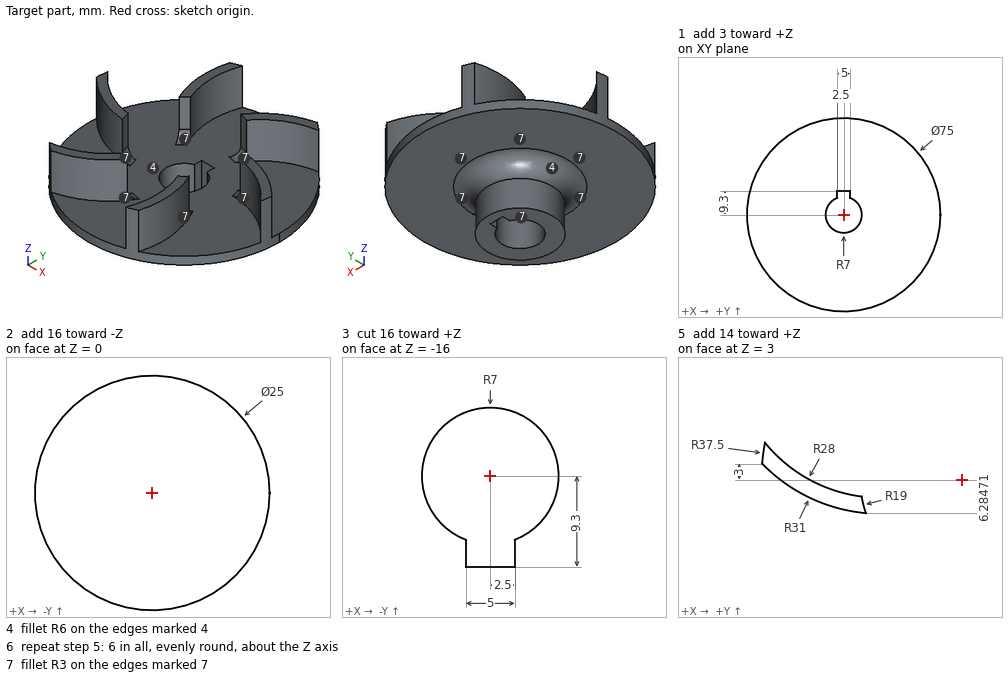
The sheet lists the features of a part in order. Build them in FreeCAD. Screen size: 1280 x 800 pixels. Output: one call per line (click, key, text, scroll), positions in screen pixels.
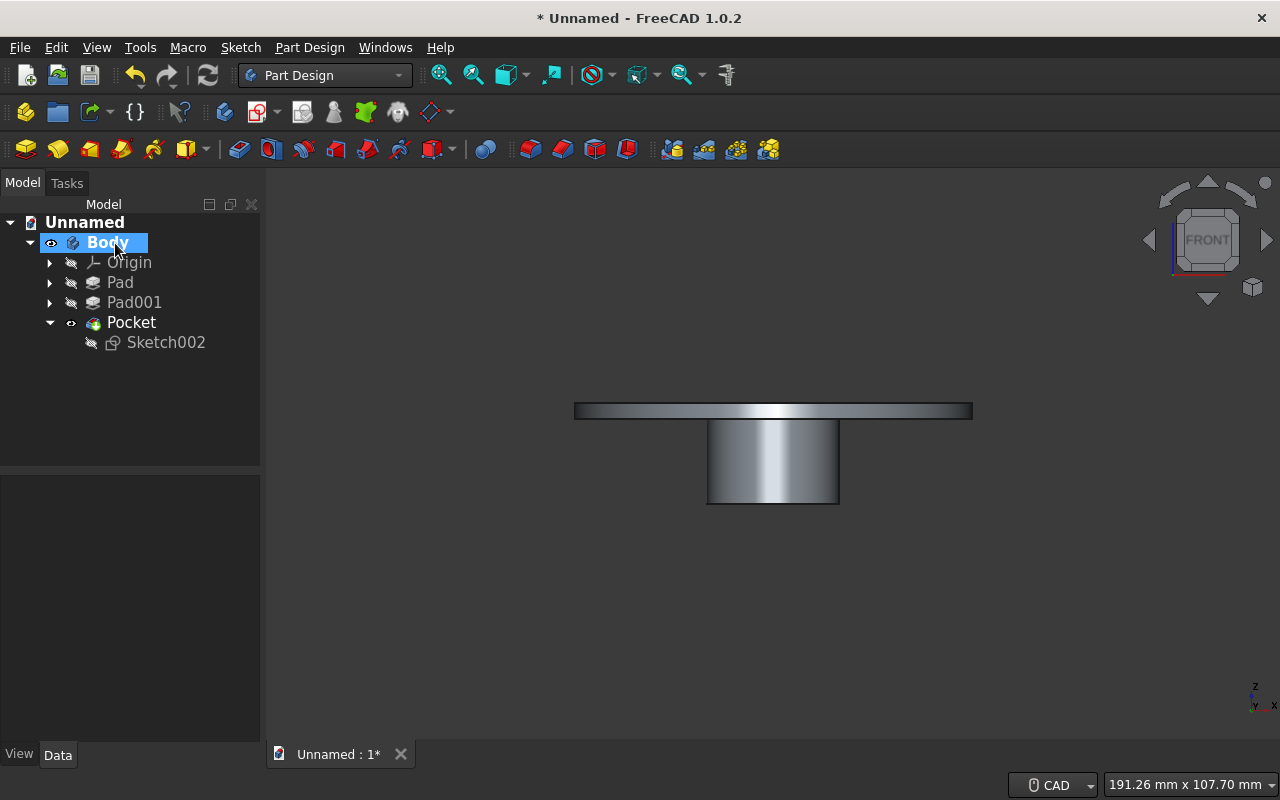
key(3)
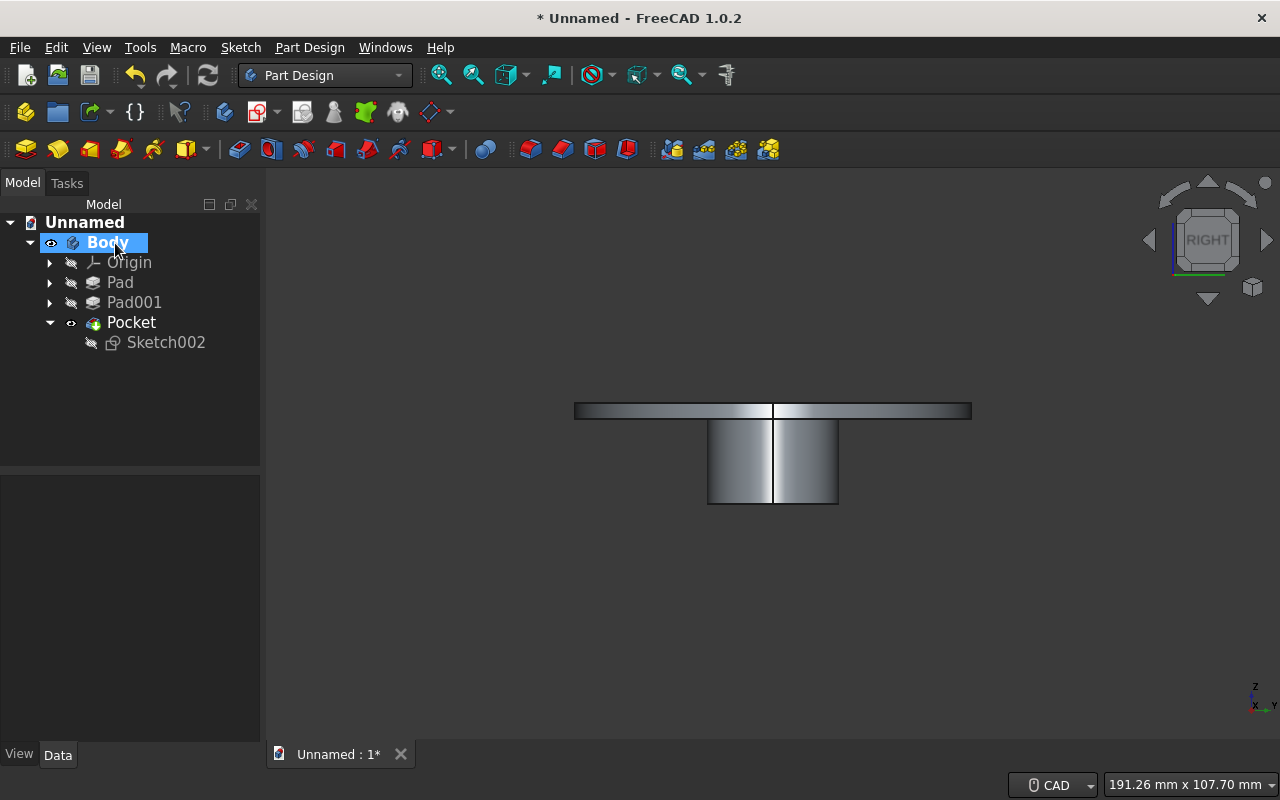
key(v)
key(f)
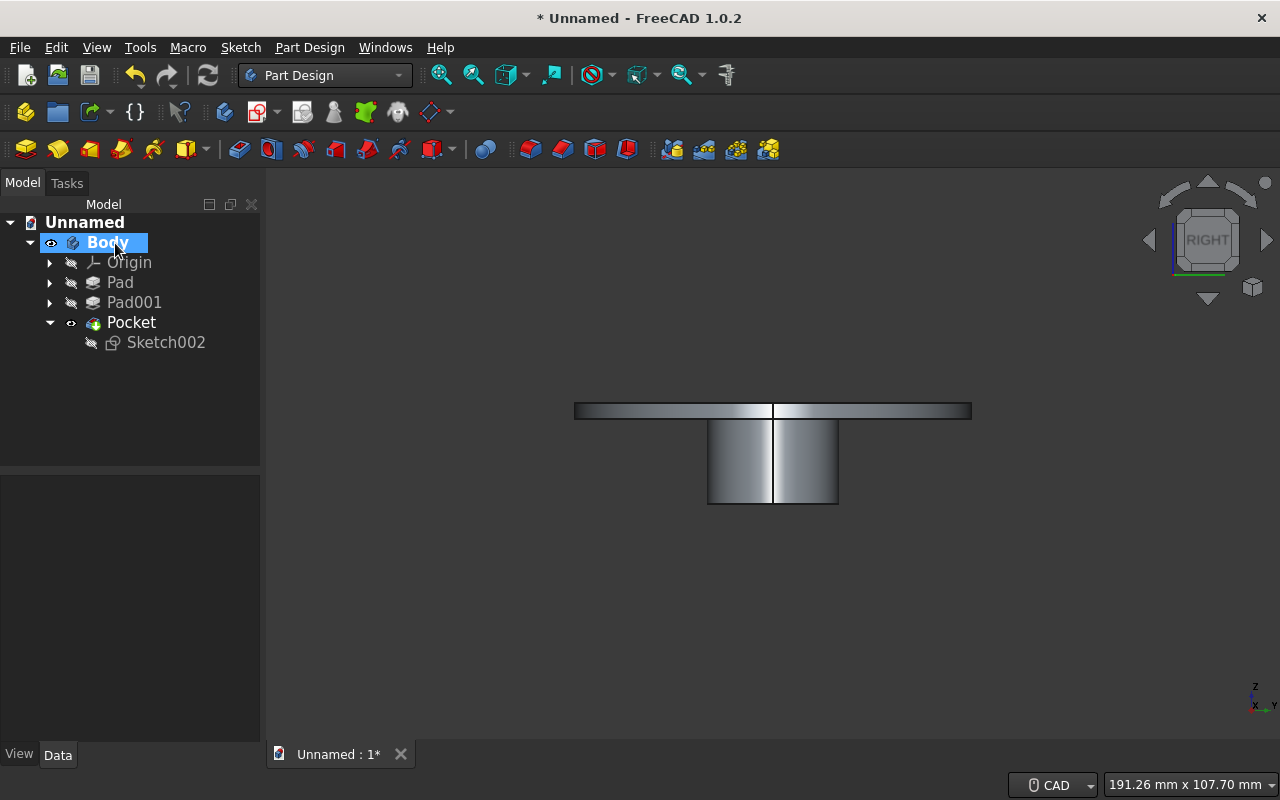
key(5)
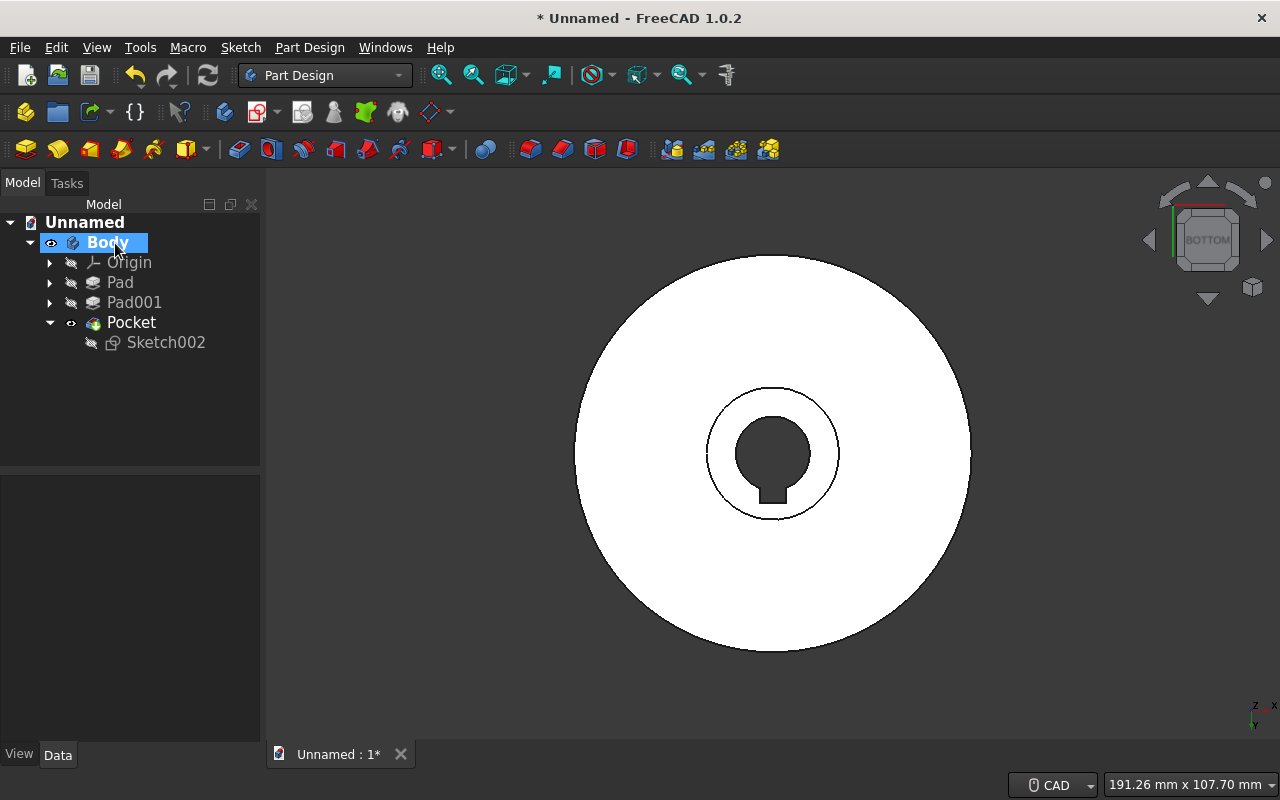
key(4)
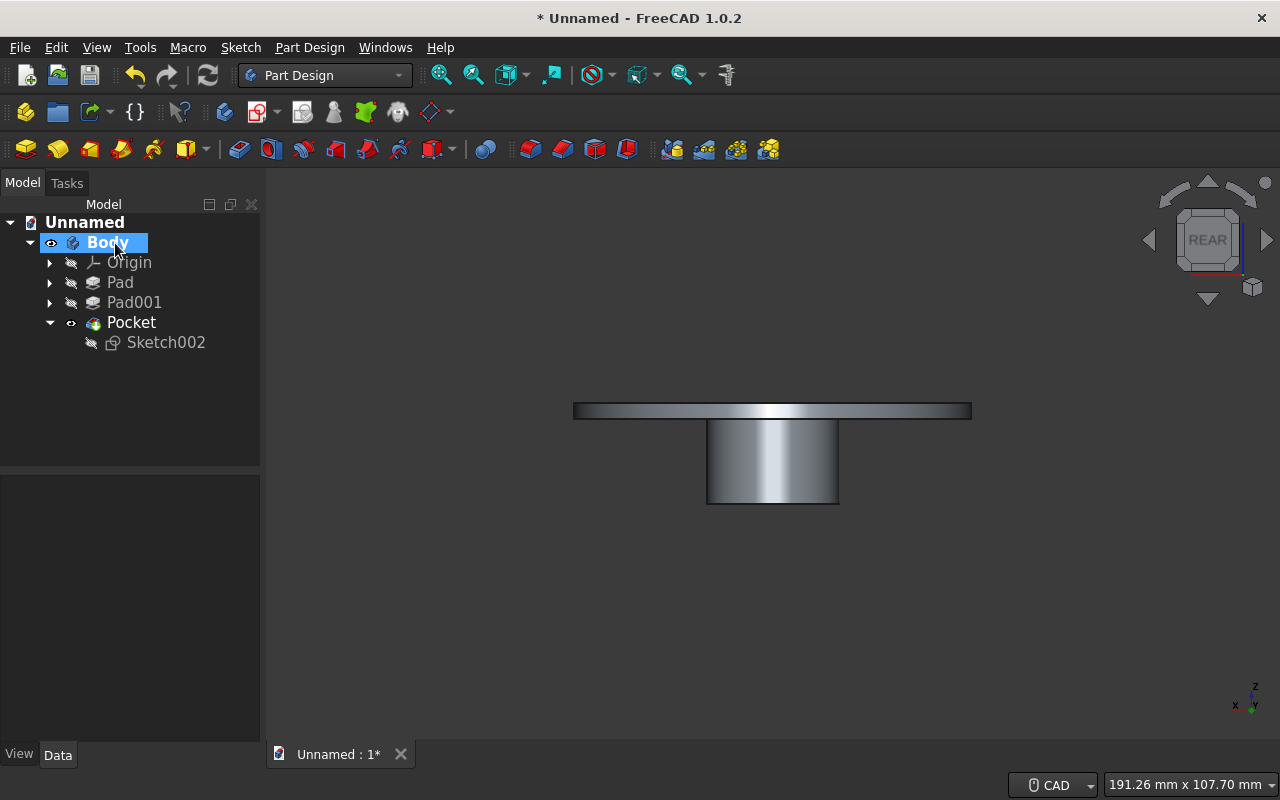
key(v)
key(f)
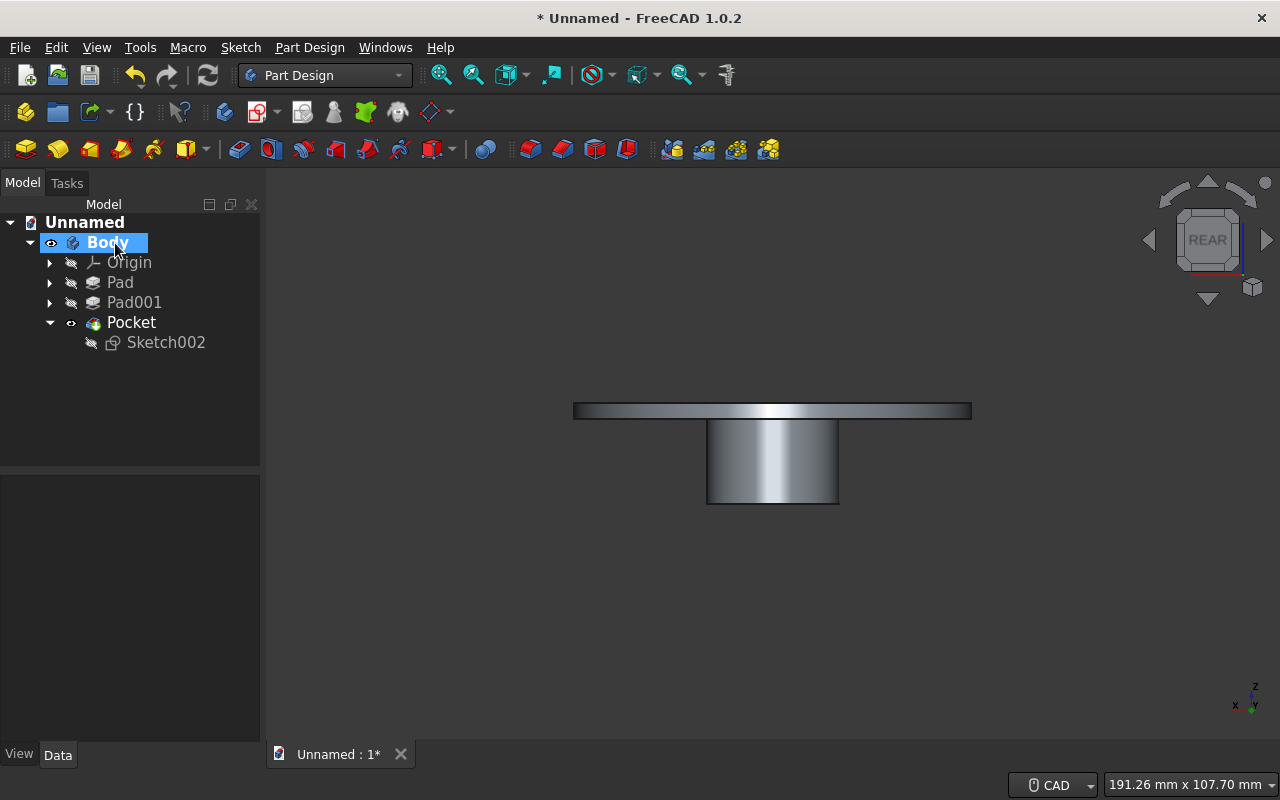
key(6)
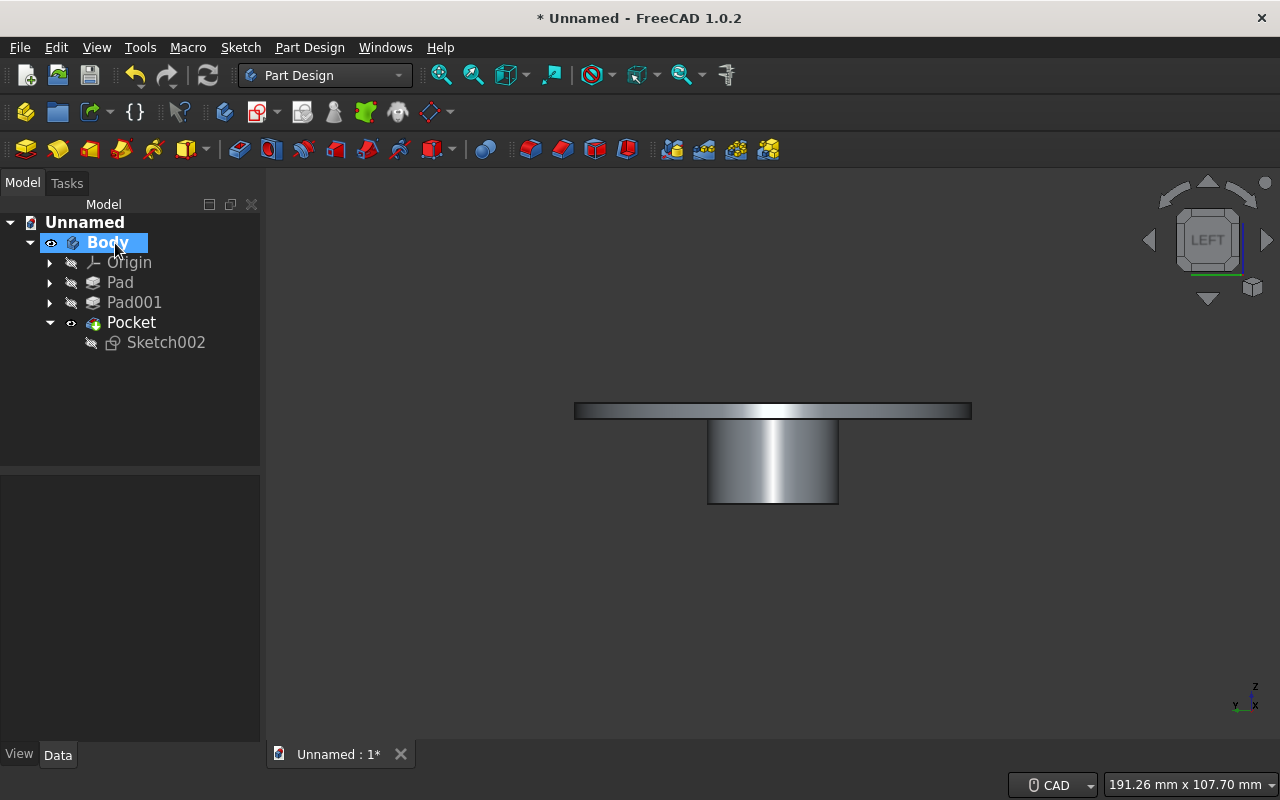
key(v)
key(f)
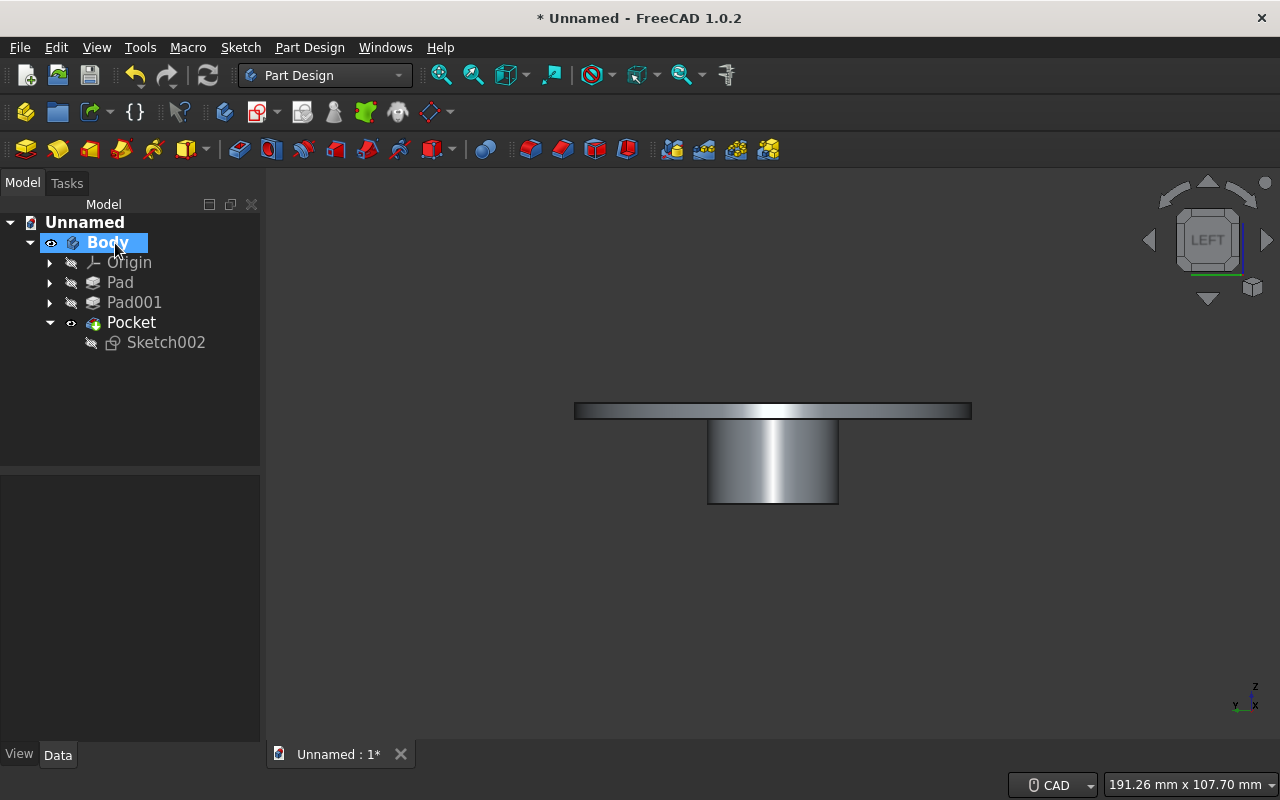
key(v)
key(3)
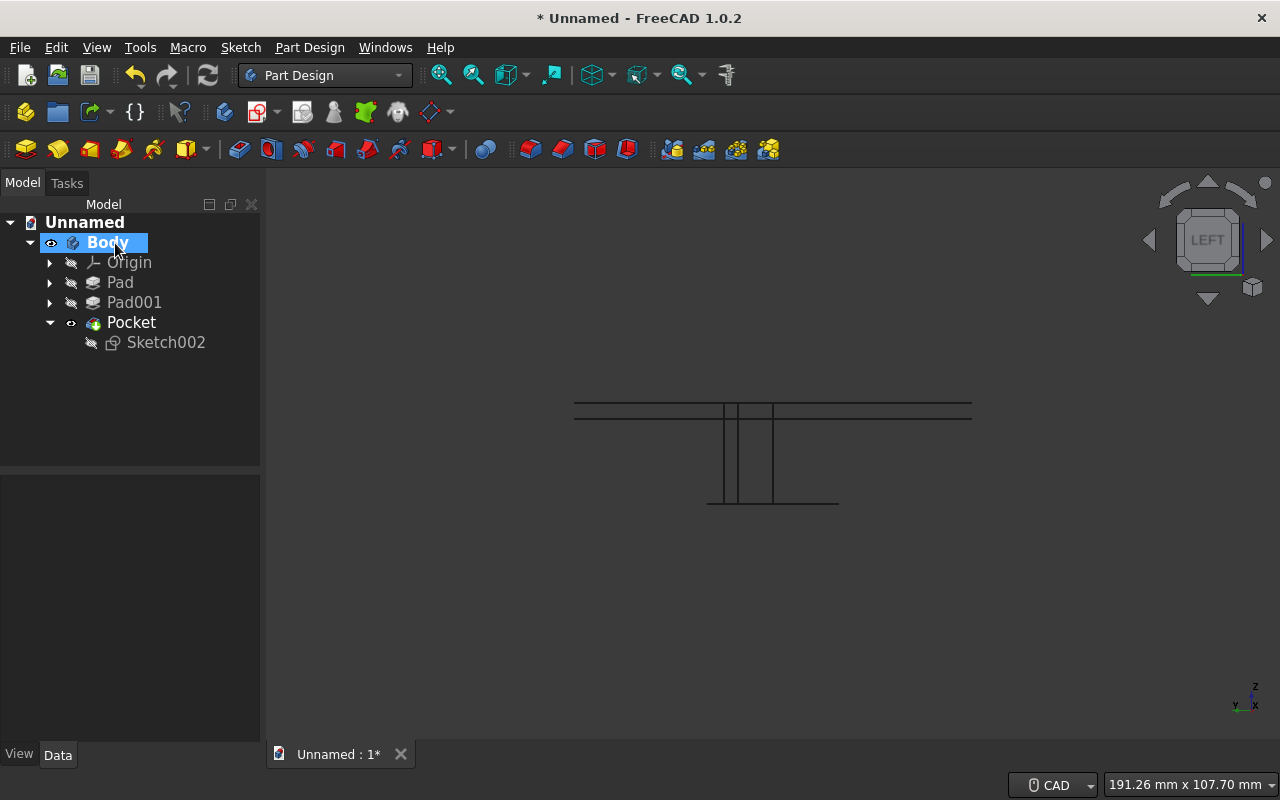
key(0)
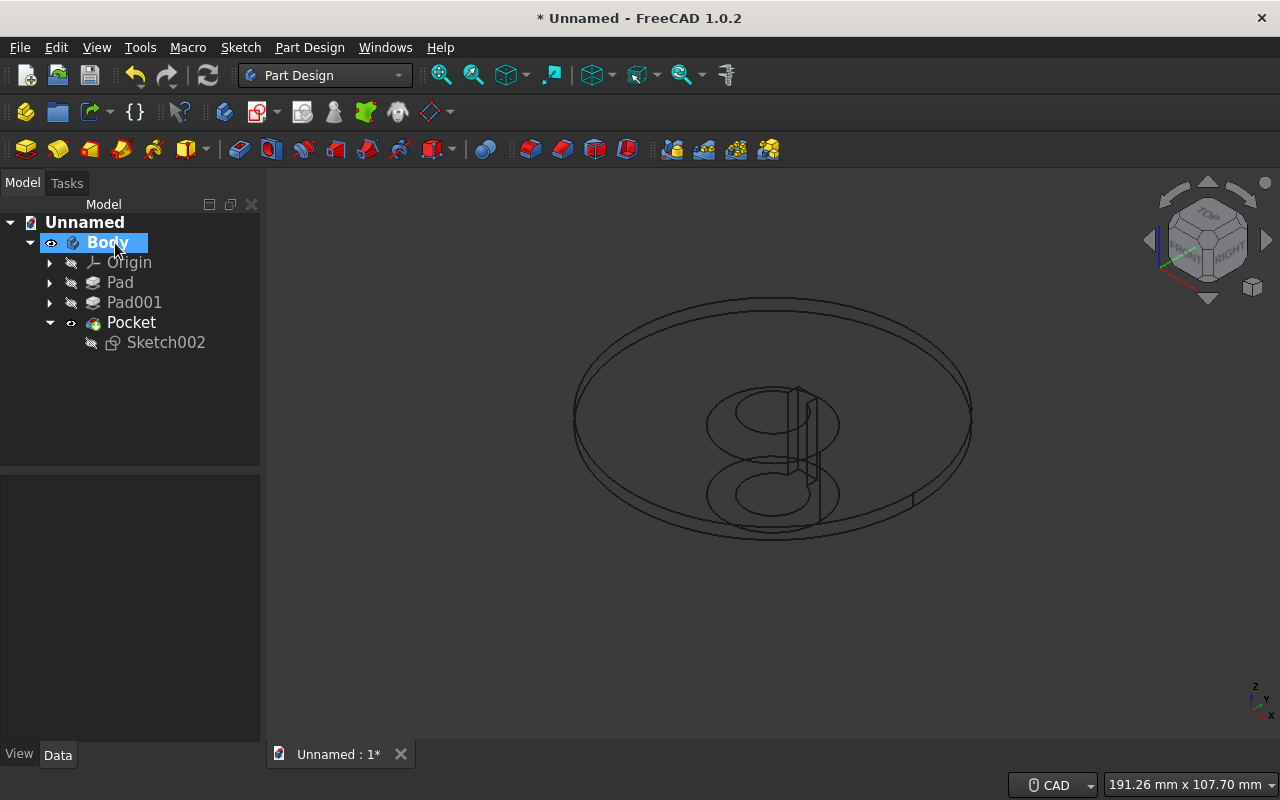
click(726, 397)